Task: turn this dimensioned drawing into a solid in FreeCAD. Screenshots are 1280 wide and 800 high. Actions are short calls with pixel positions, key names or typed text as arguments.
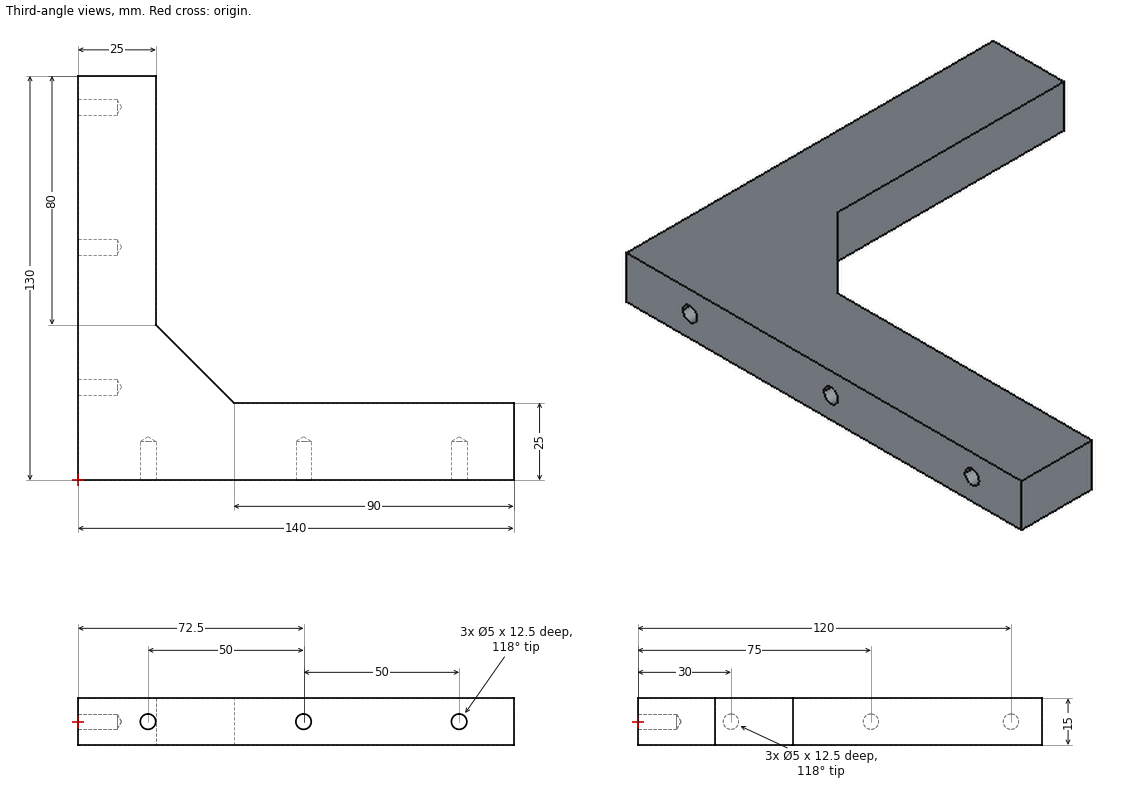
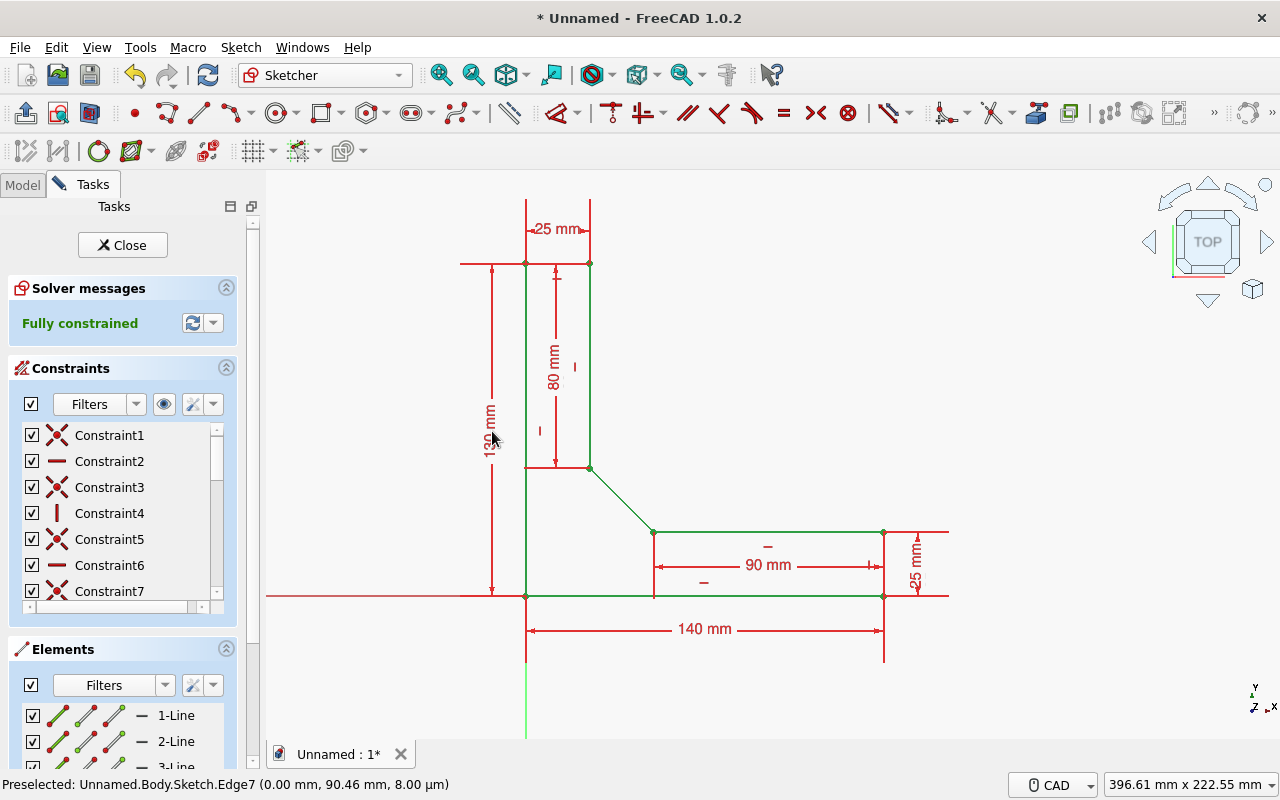
click(123, 245)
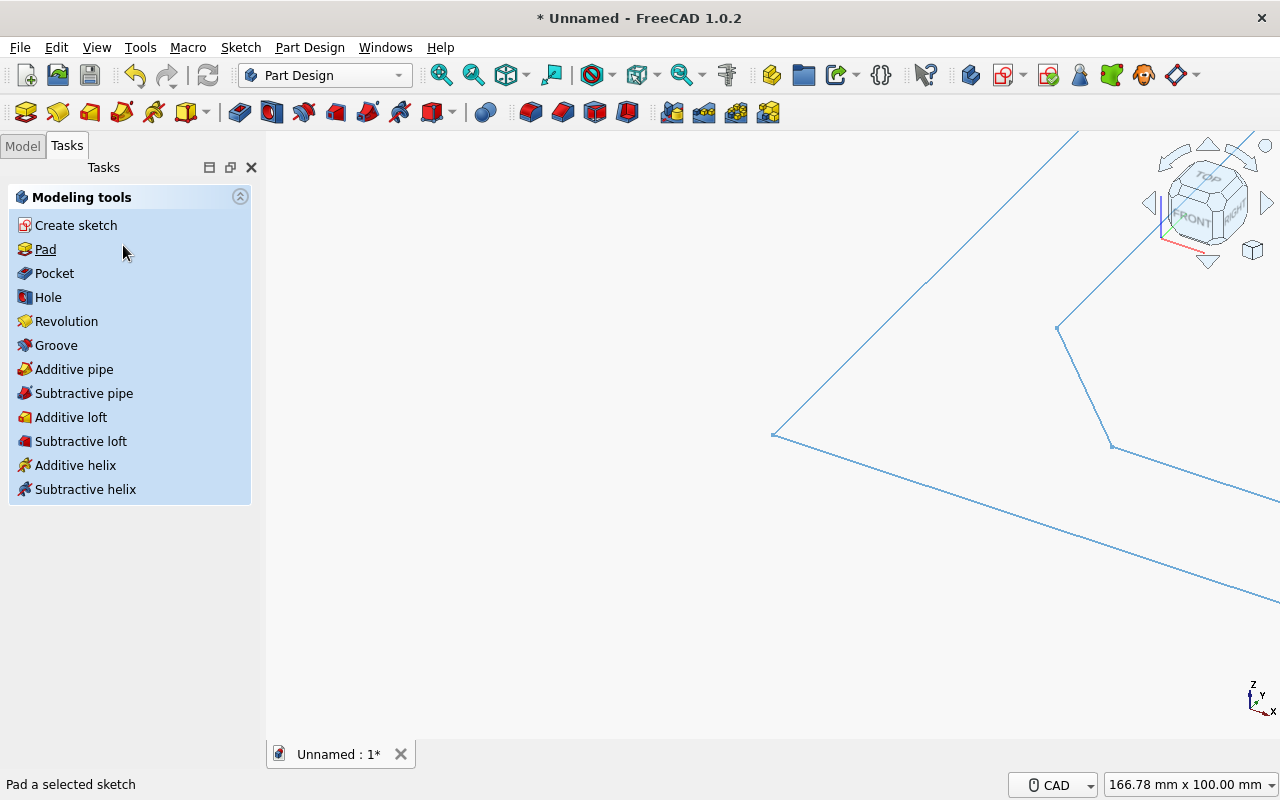
click(26, 112)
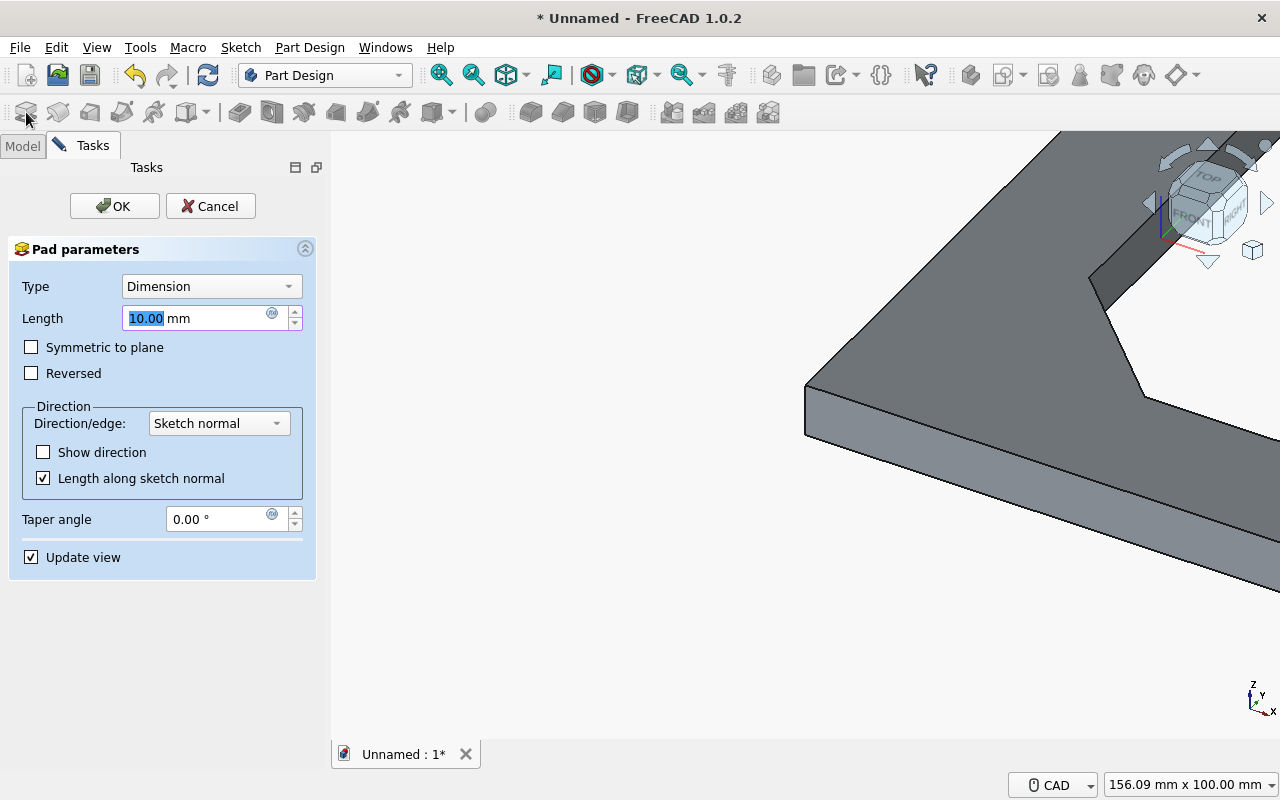
text(15)
key(Tab)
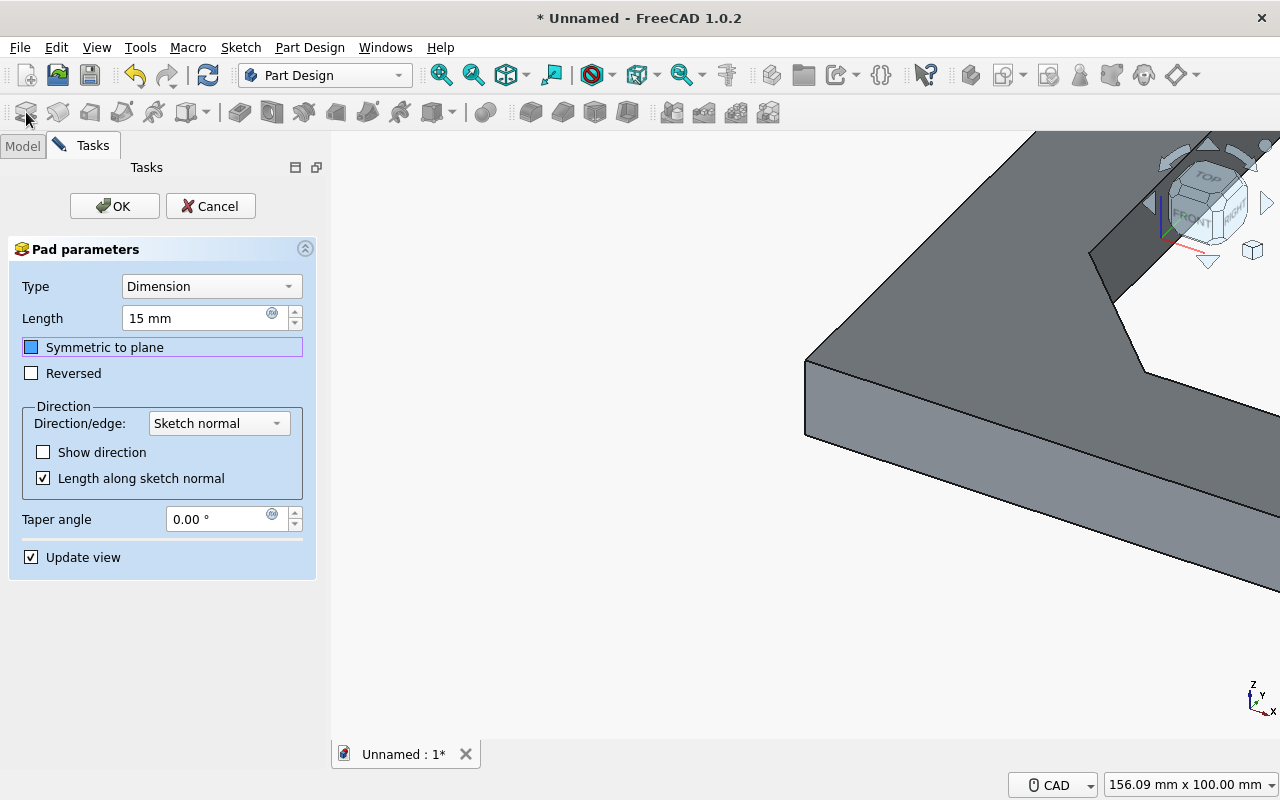
click(30, 347)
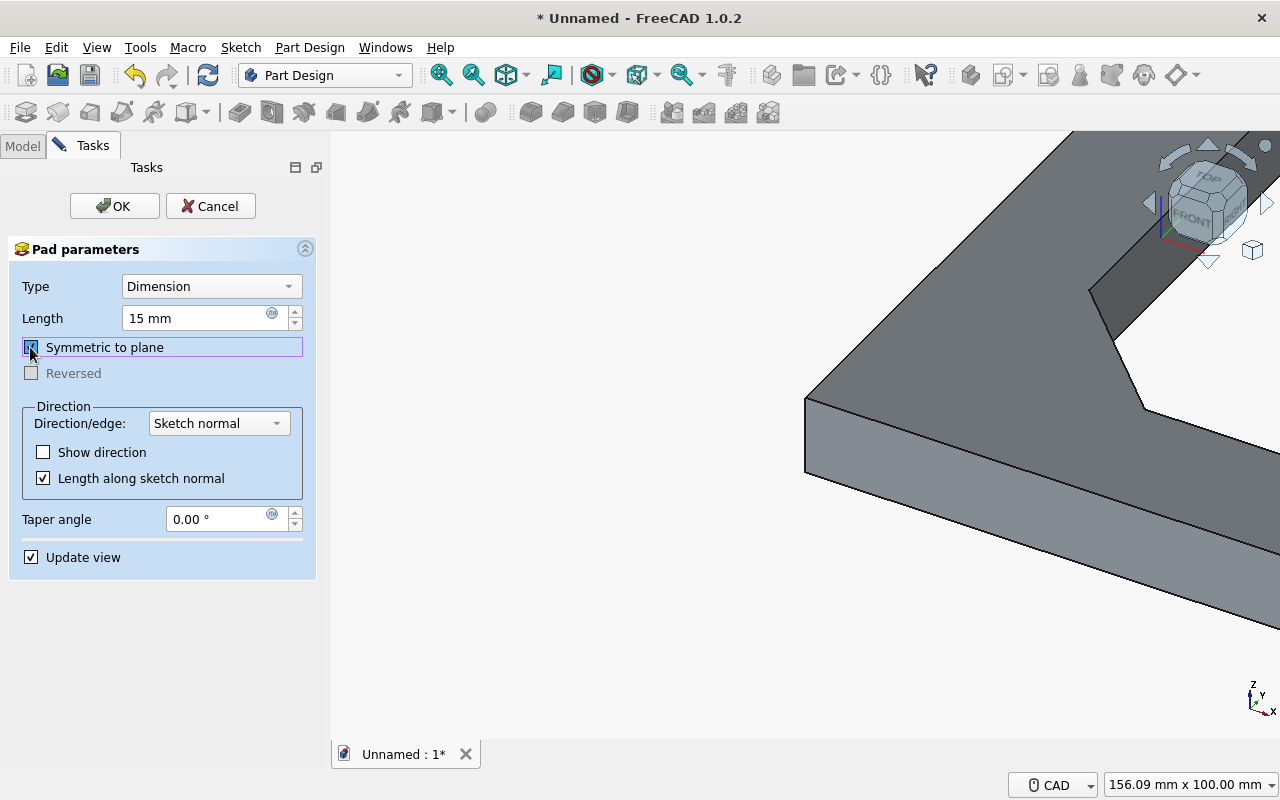
click(115, 206)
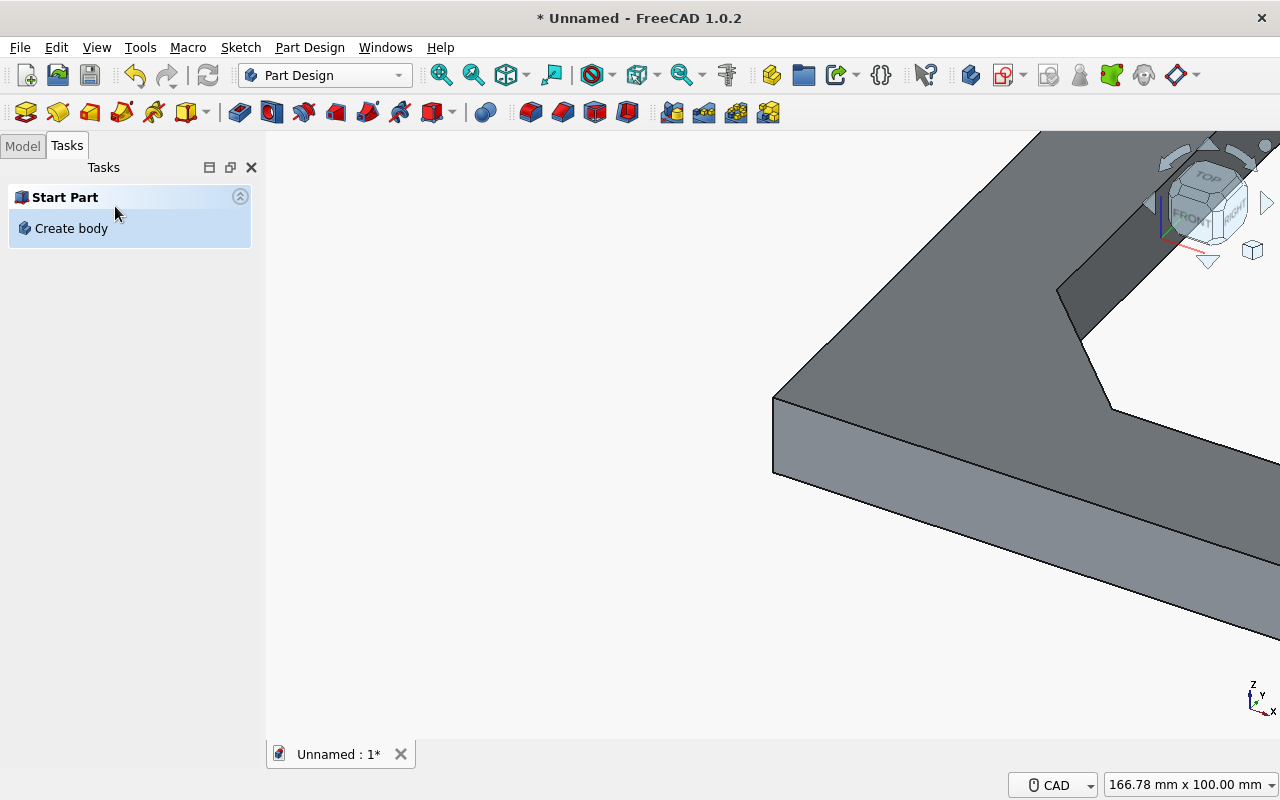
click(442, 76)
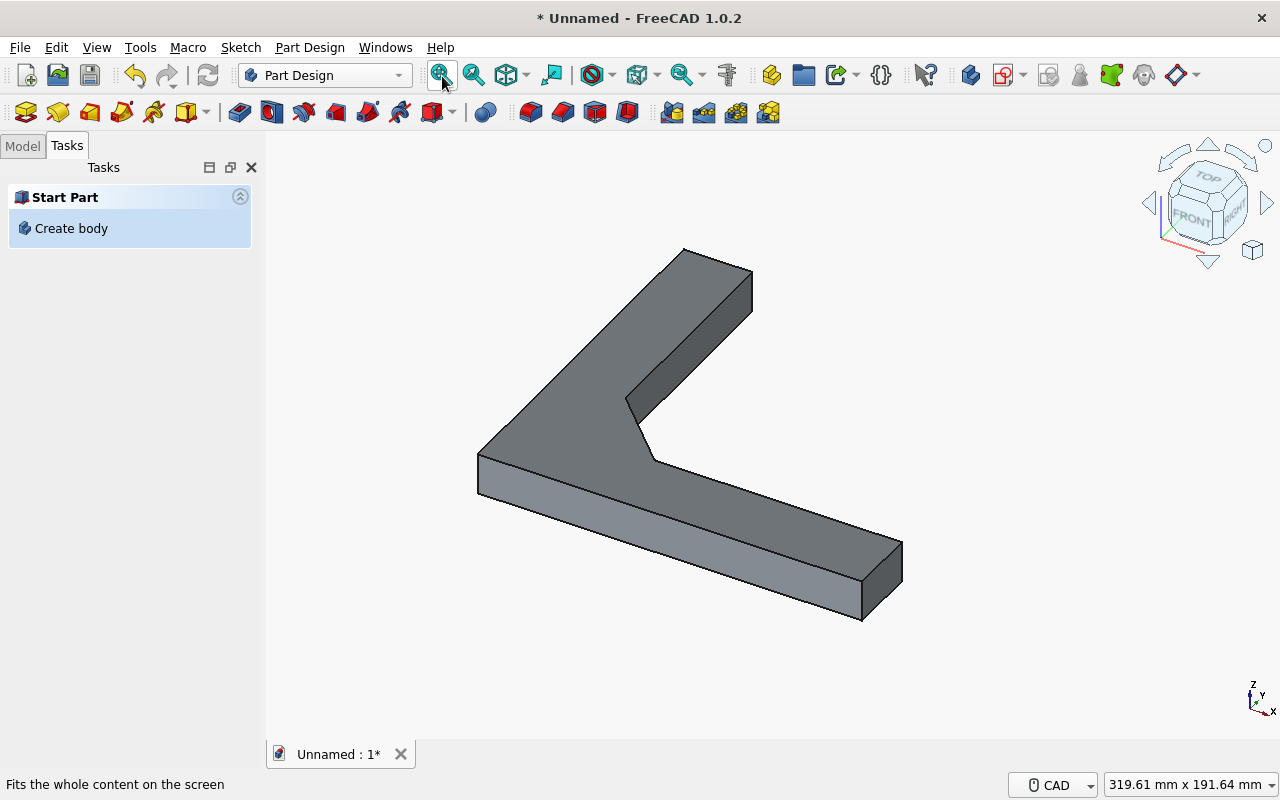
click(1004, 76)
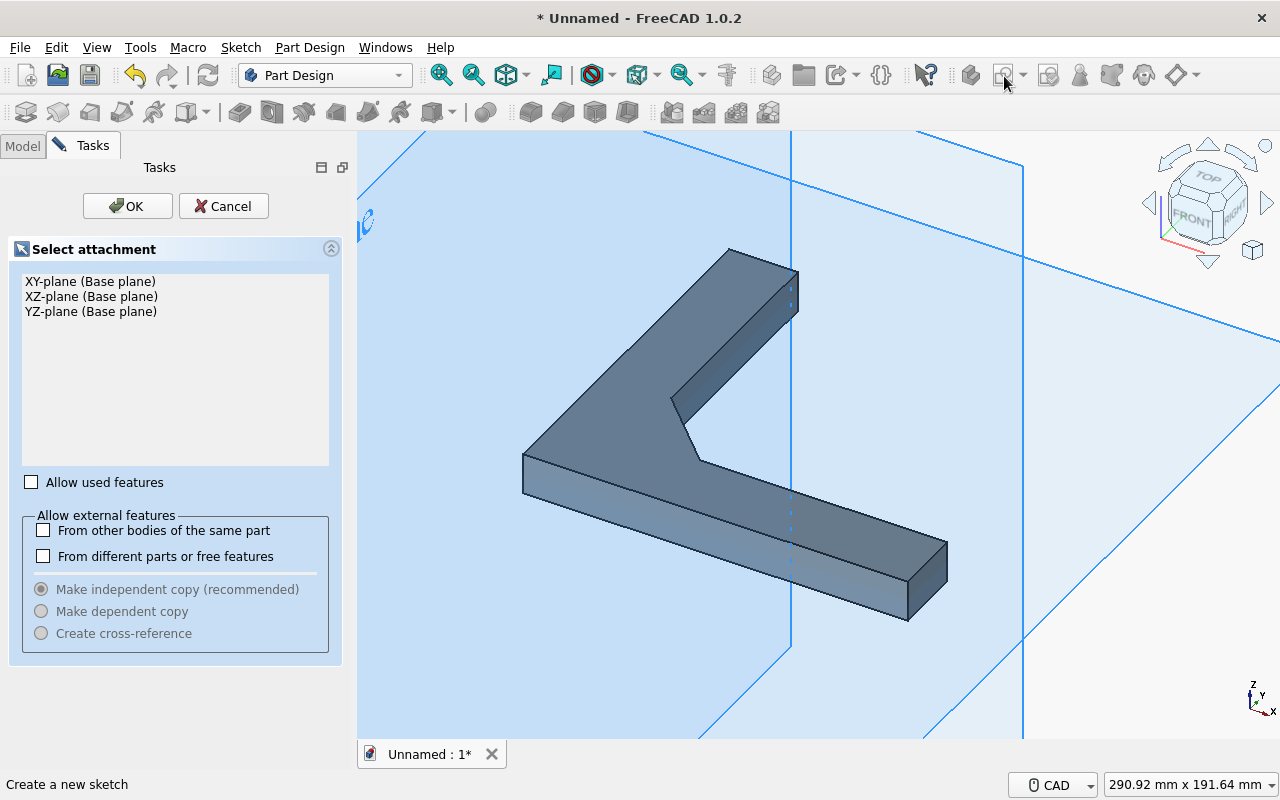
click(82, 296)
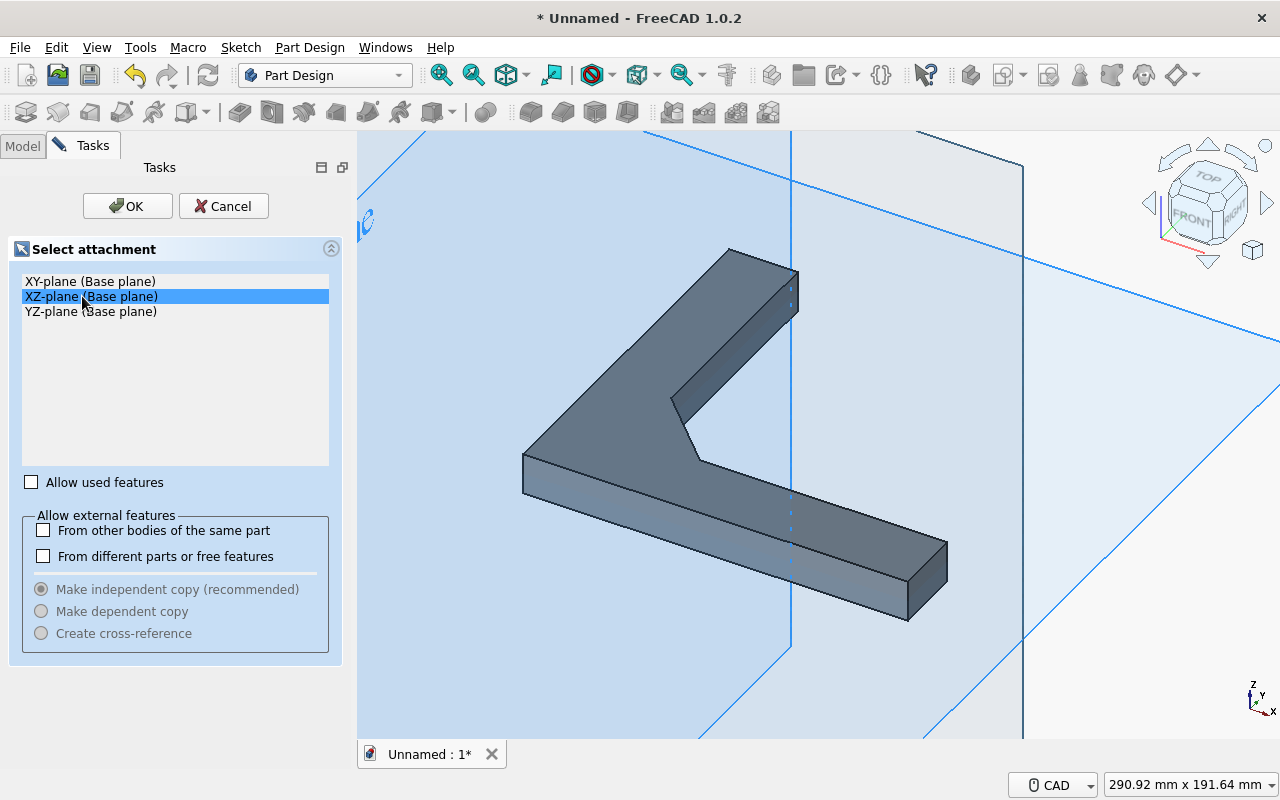
click(128, 206)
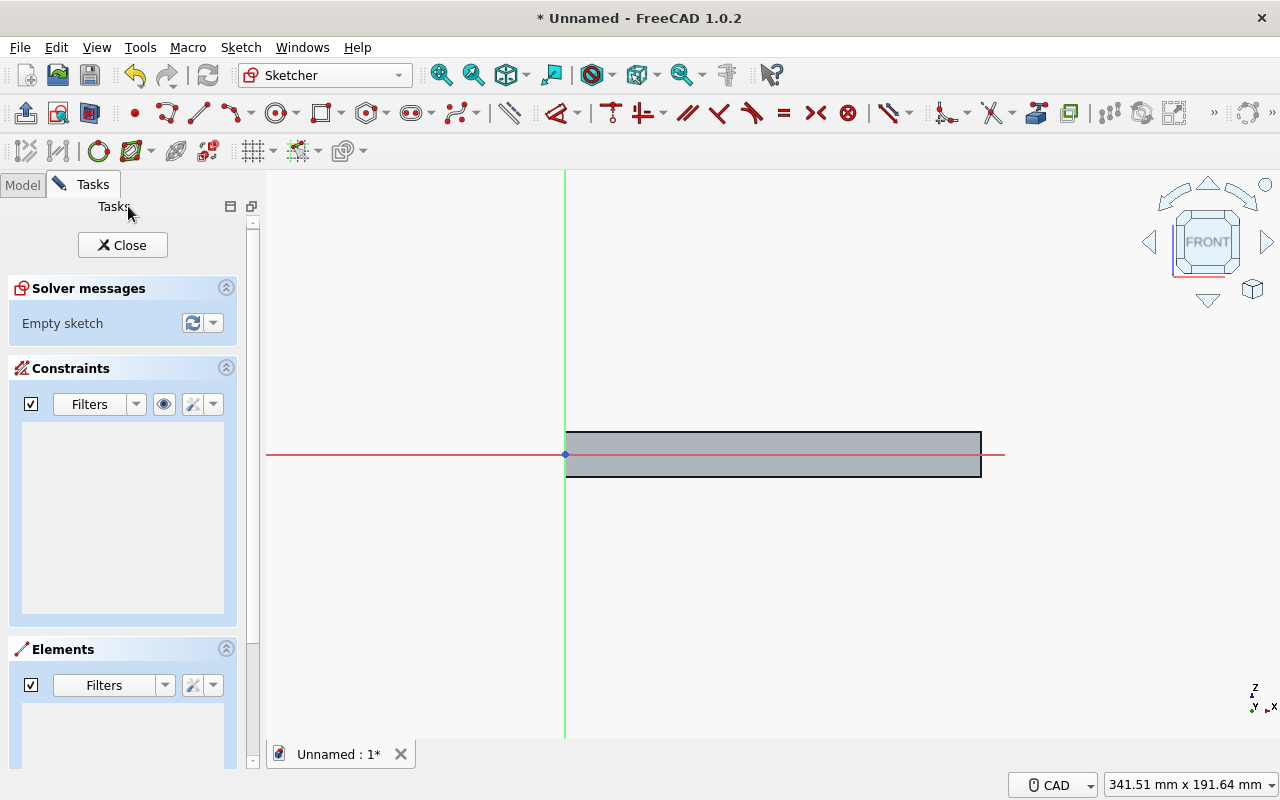
scroll(845, 455, up, 2)